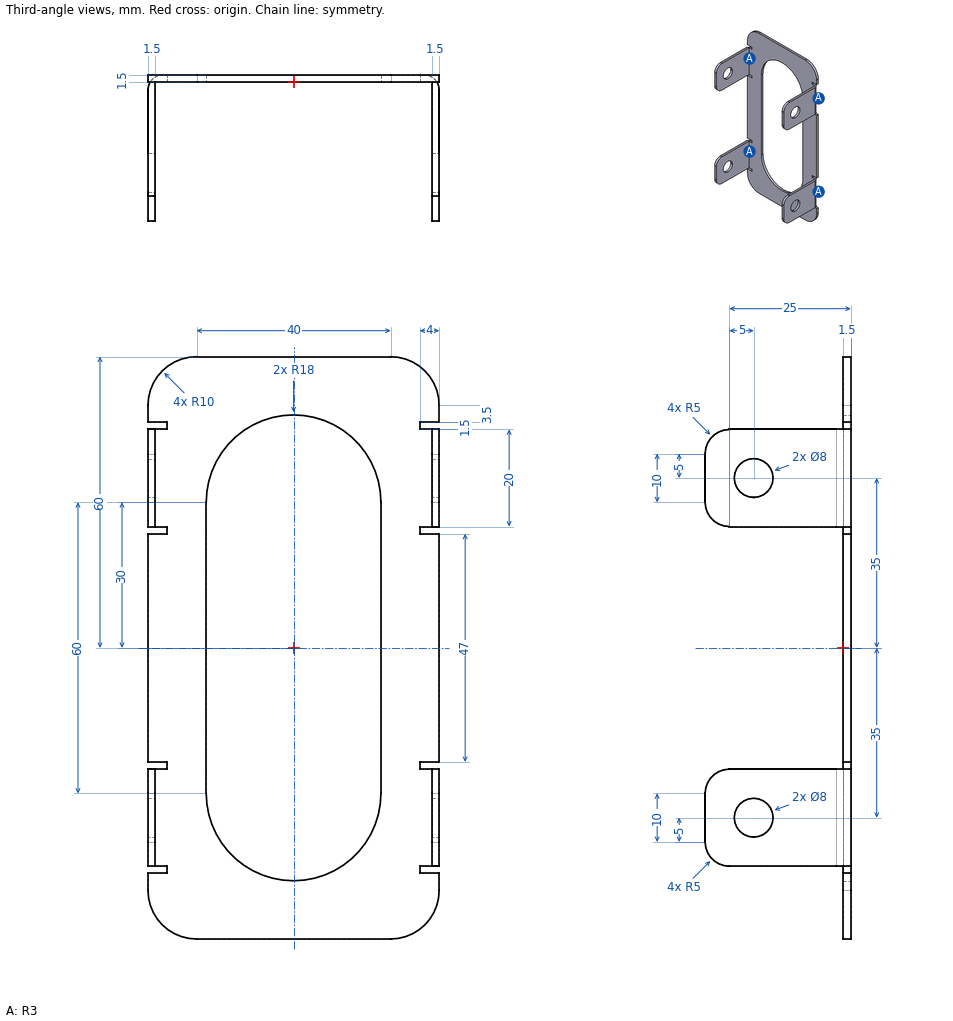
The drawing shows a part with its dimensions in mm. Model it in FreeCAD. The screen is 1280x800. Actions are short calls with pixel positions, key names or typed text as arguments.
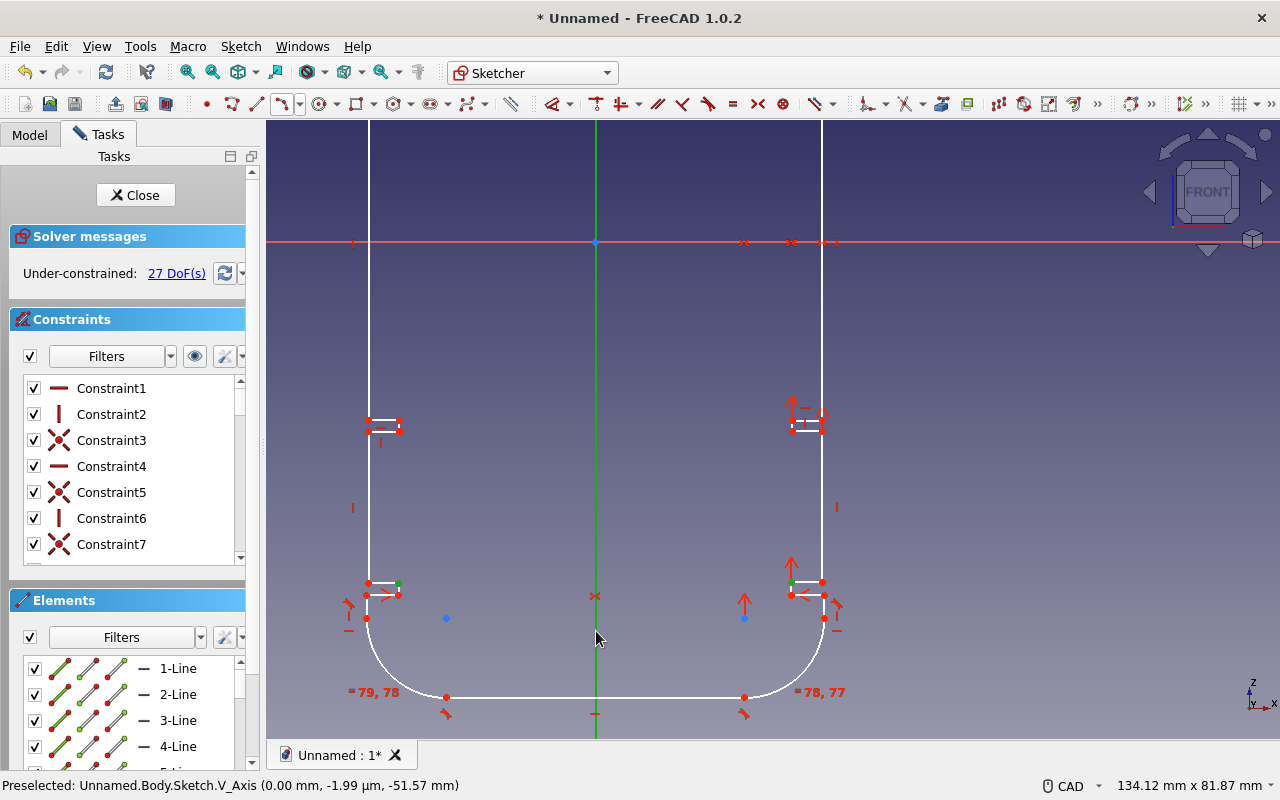
click(758, 104)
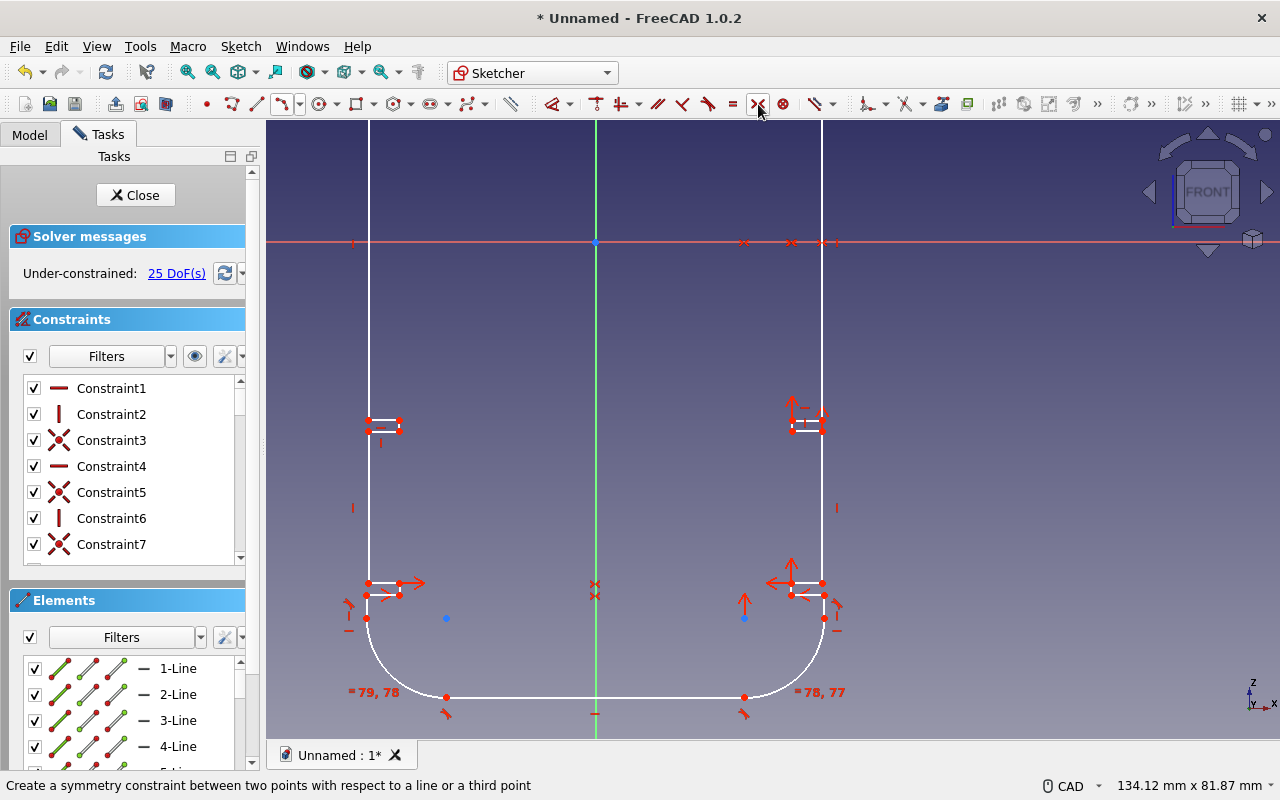
click(822, 431)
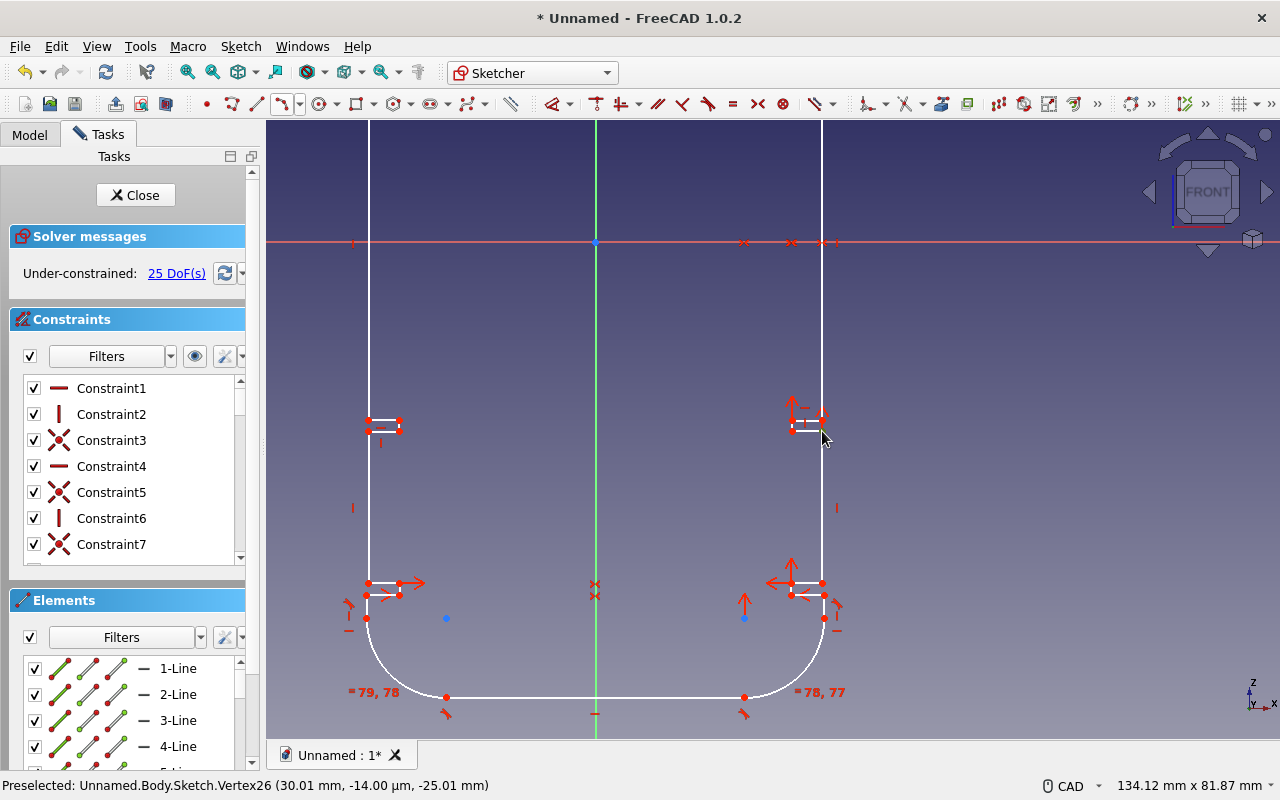
click(369, 432)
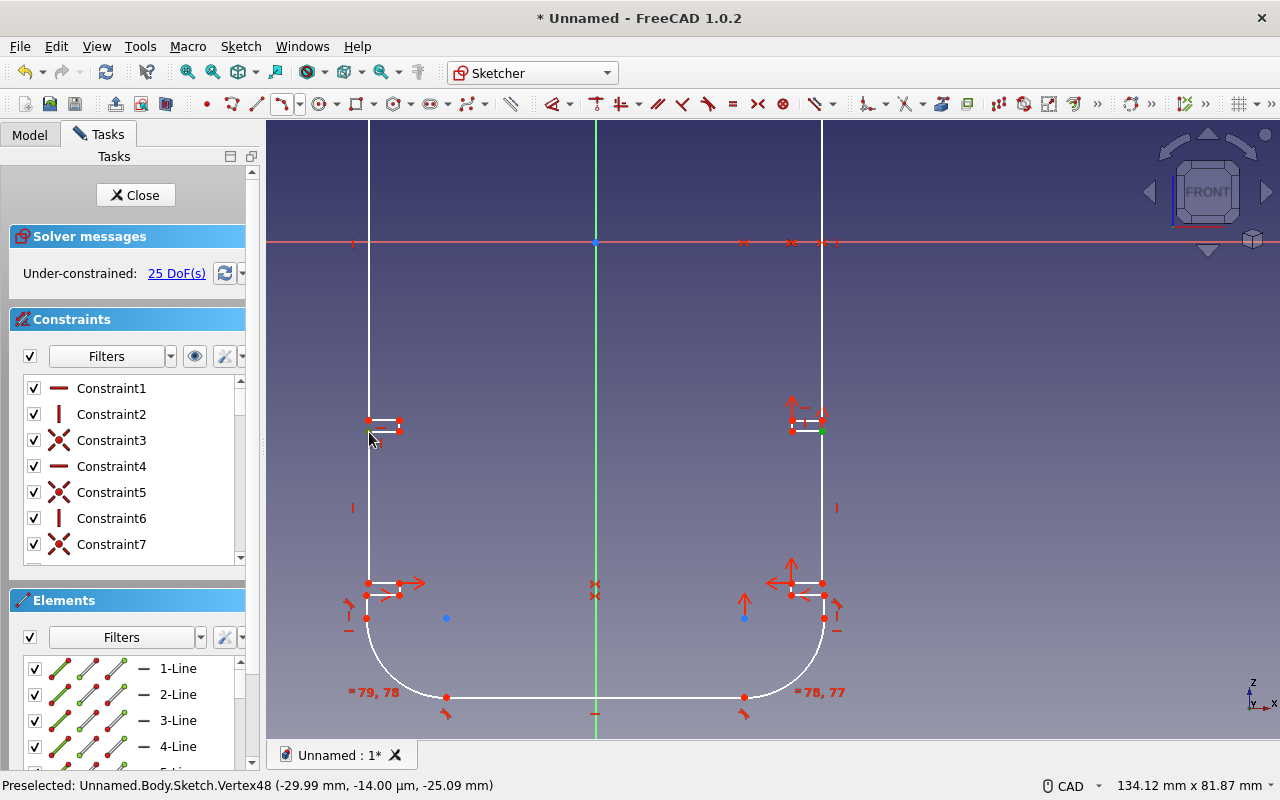
click(596, 631)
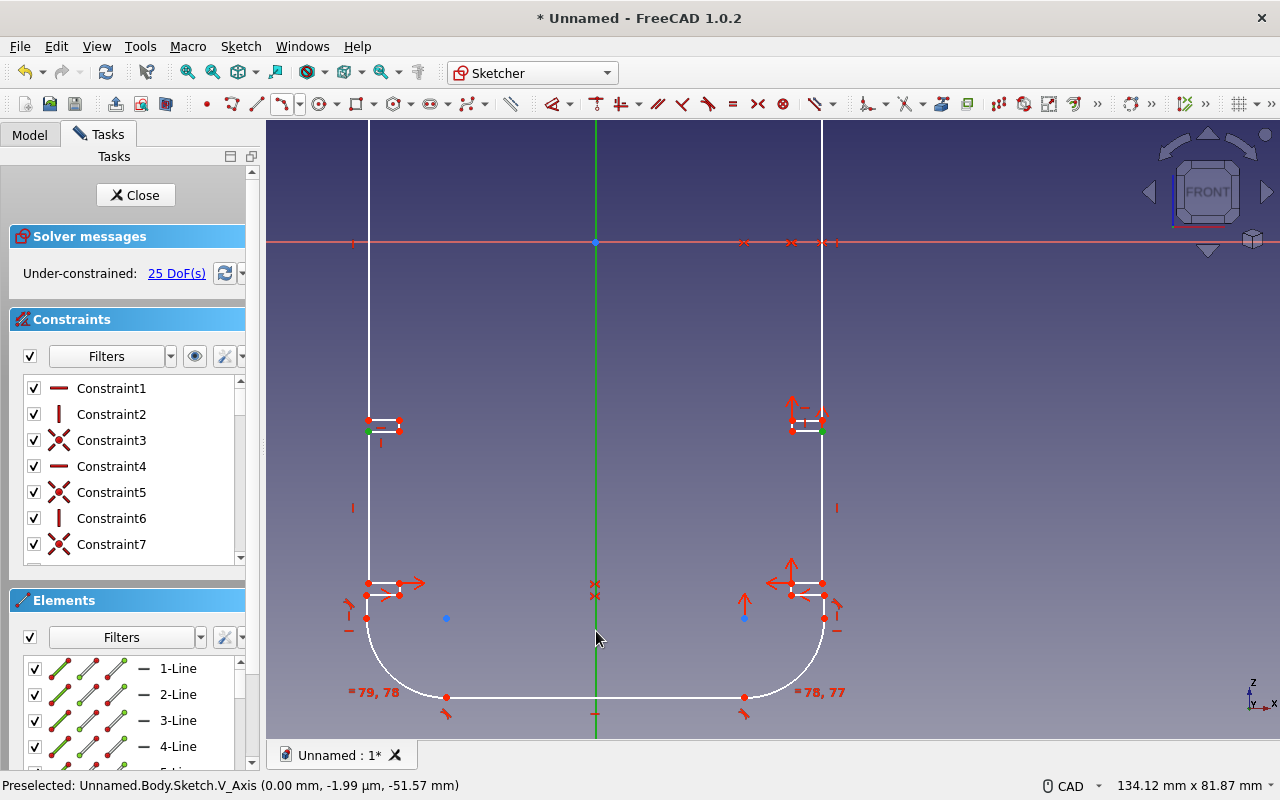
click(758, 104)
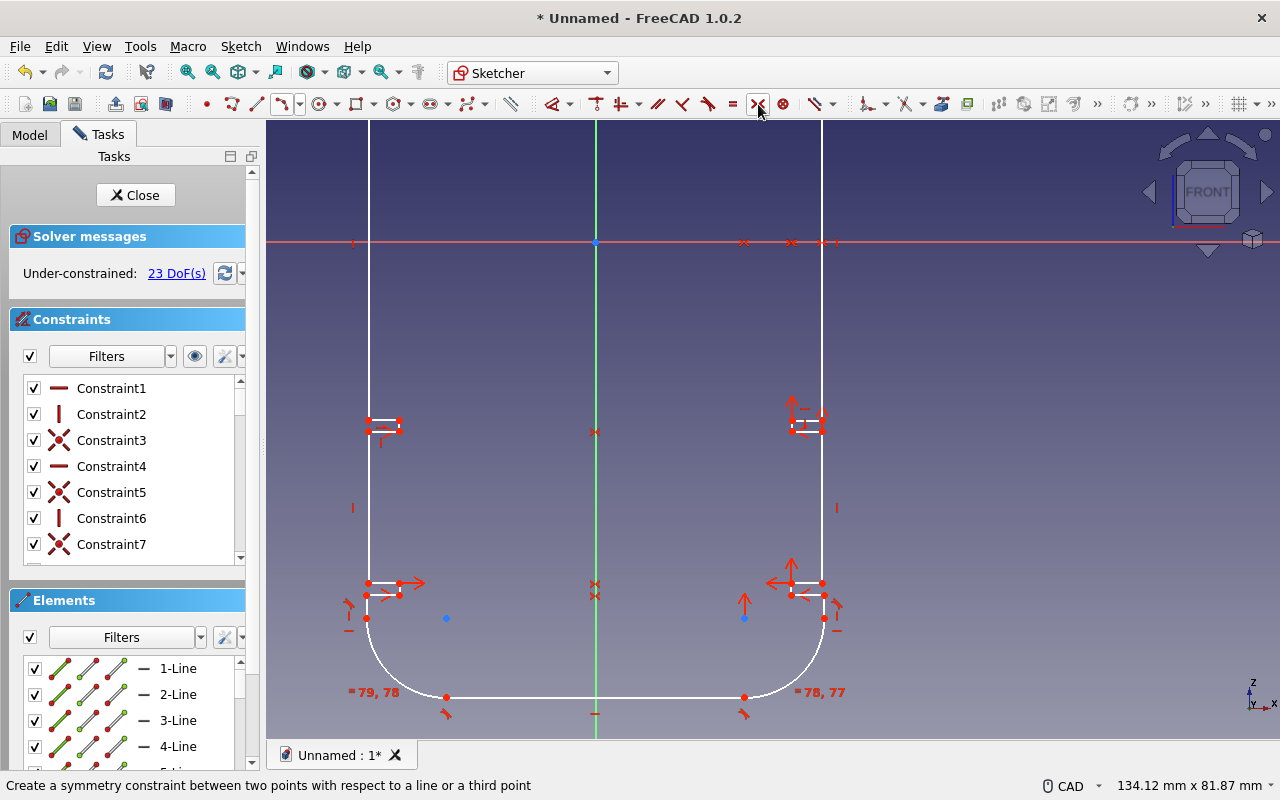
click(792, 421)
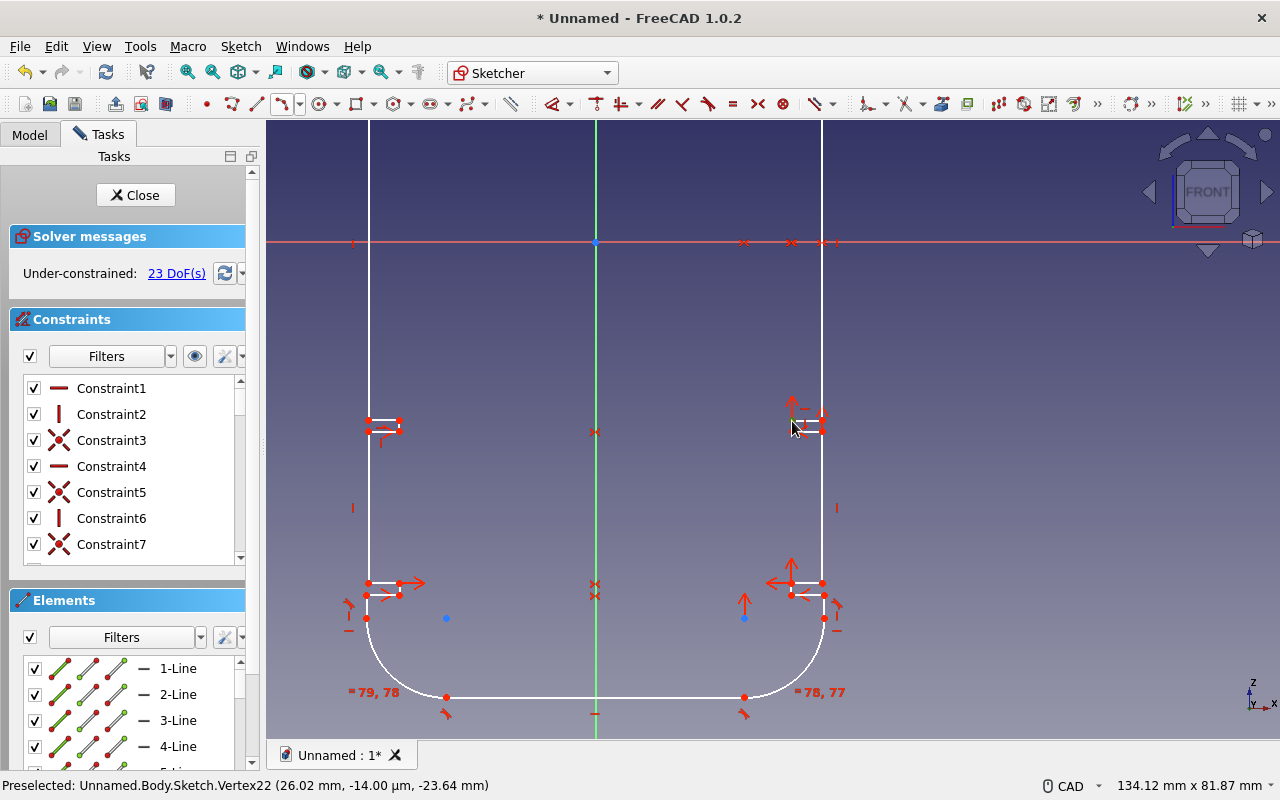
click(399, 420)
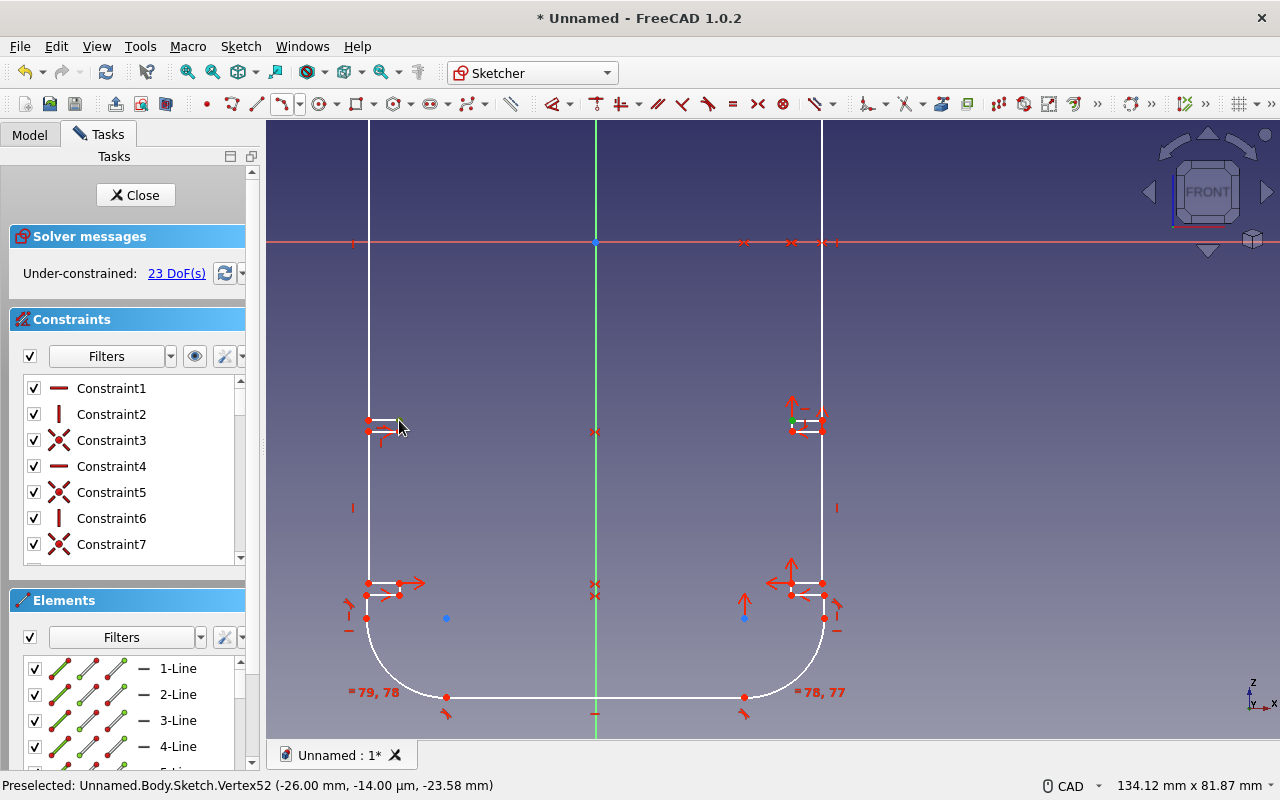
click(596, 631)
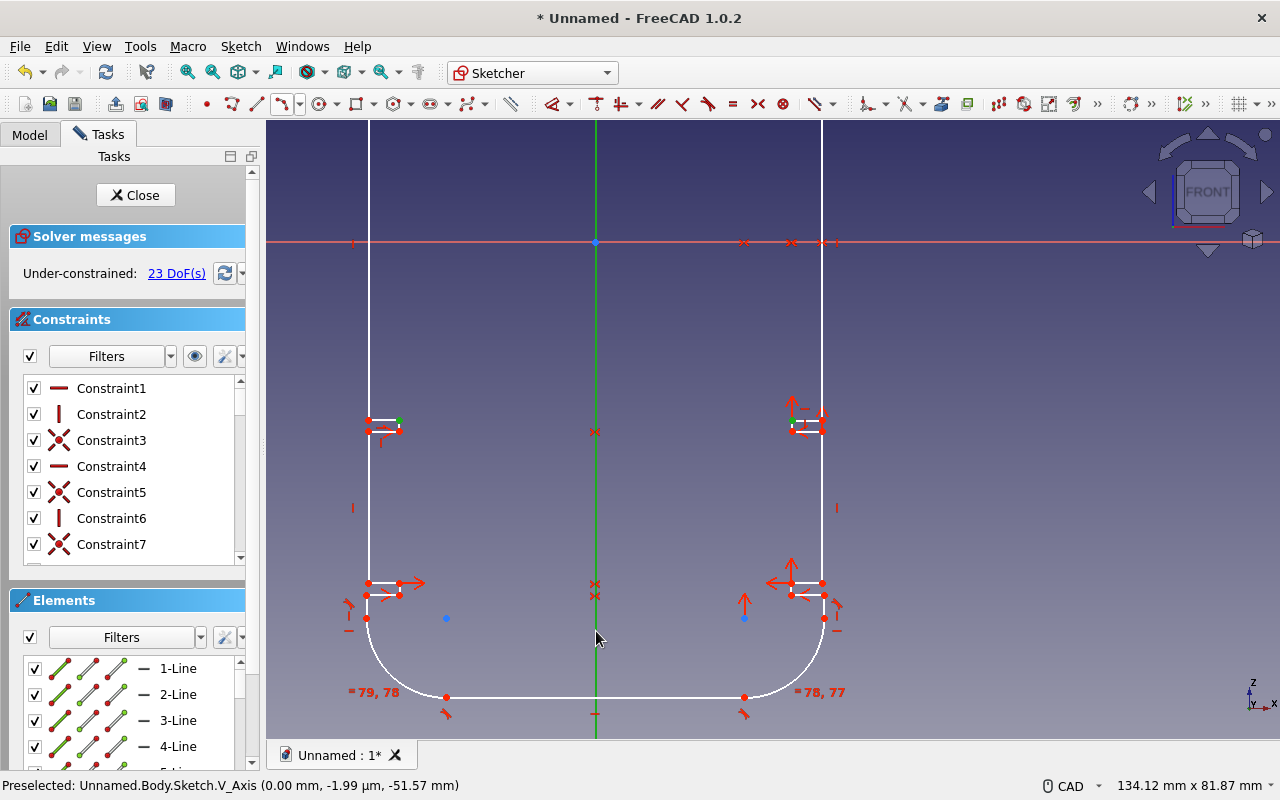
key(s)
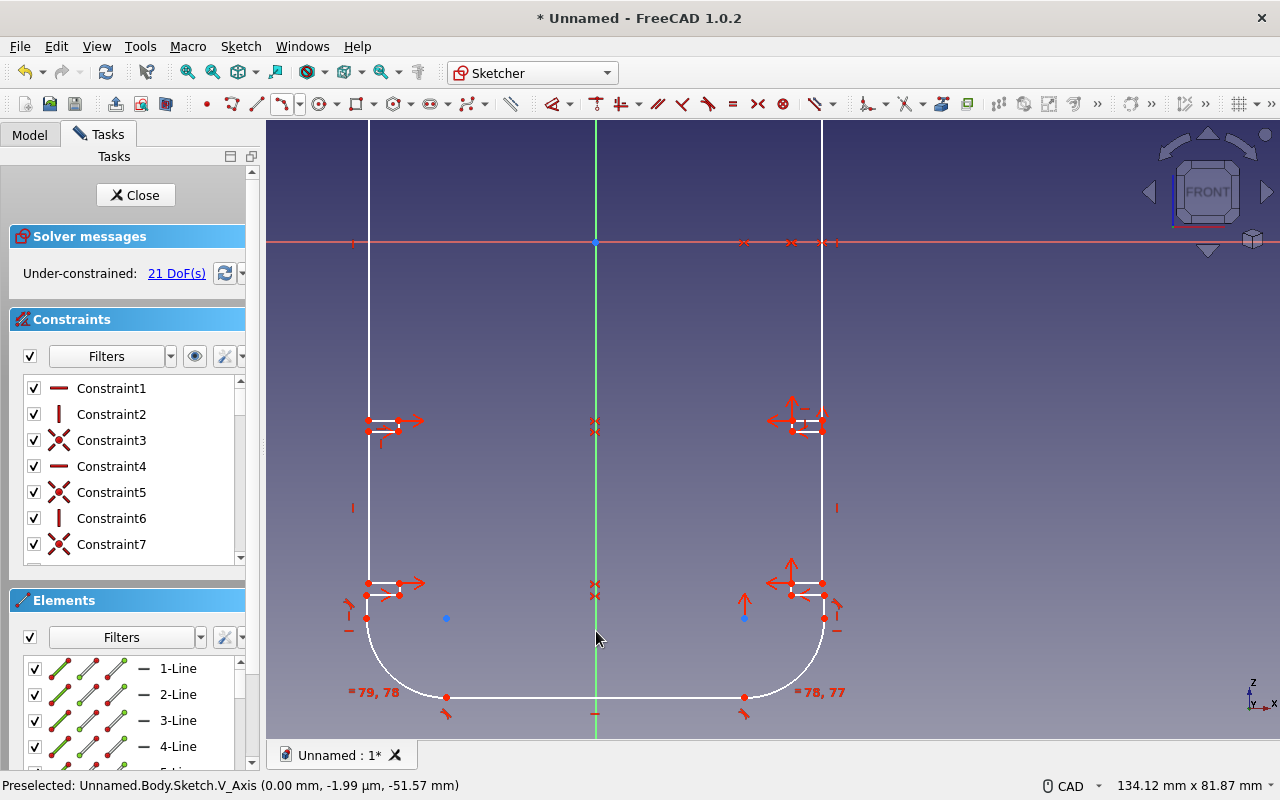
scroll(793, 582, down, 4)